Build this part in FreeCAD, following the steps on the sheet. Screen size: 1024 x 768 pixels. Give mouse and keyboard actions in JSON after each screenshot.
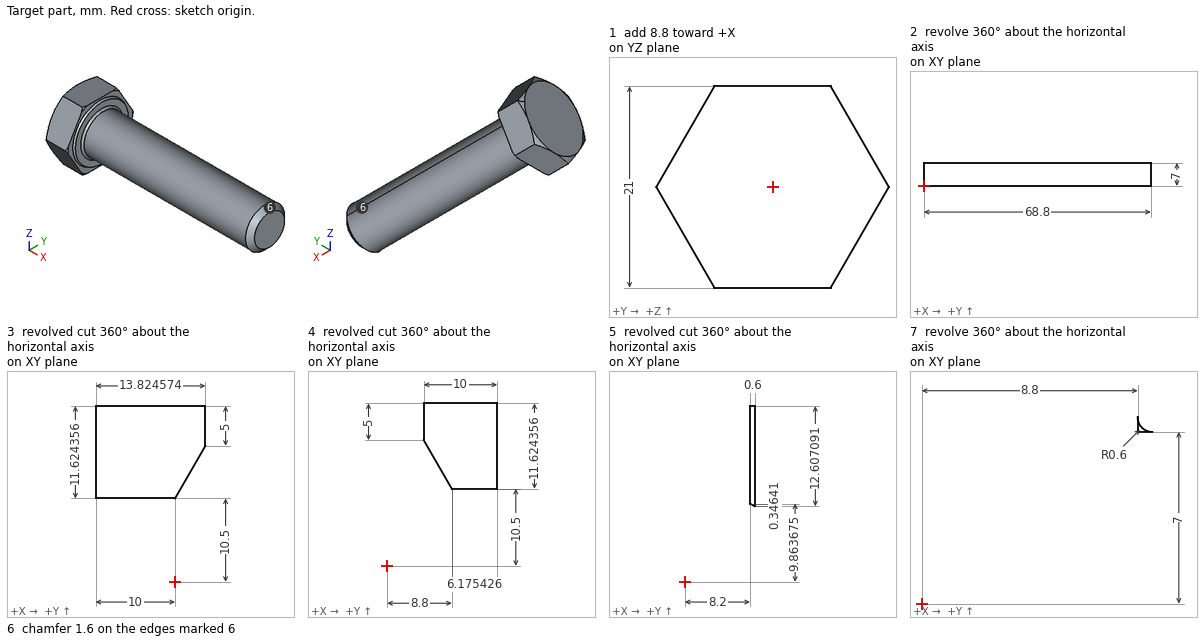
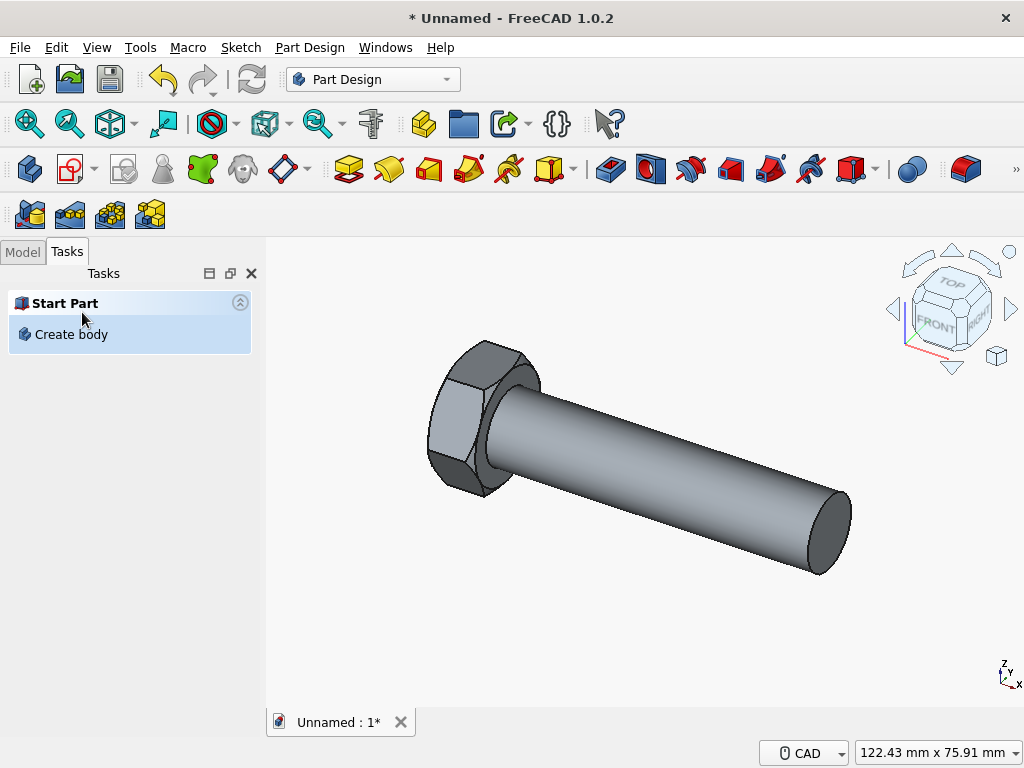
{"action": "left_click", "coordinate": [70, 170]}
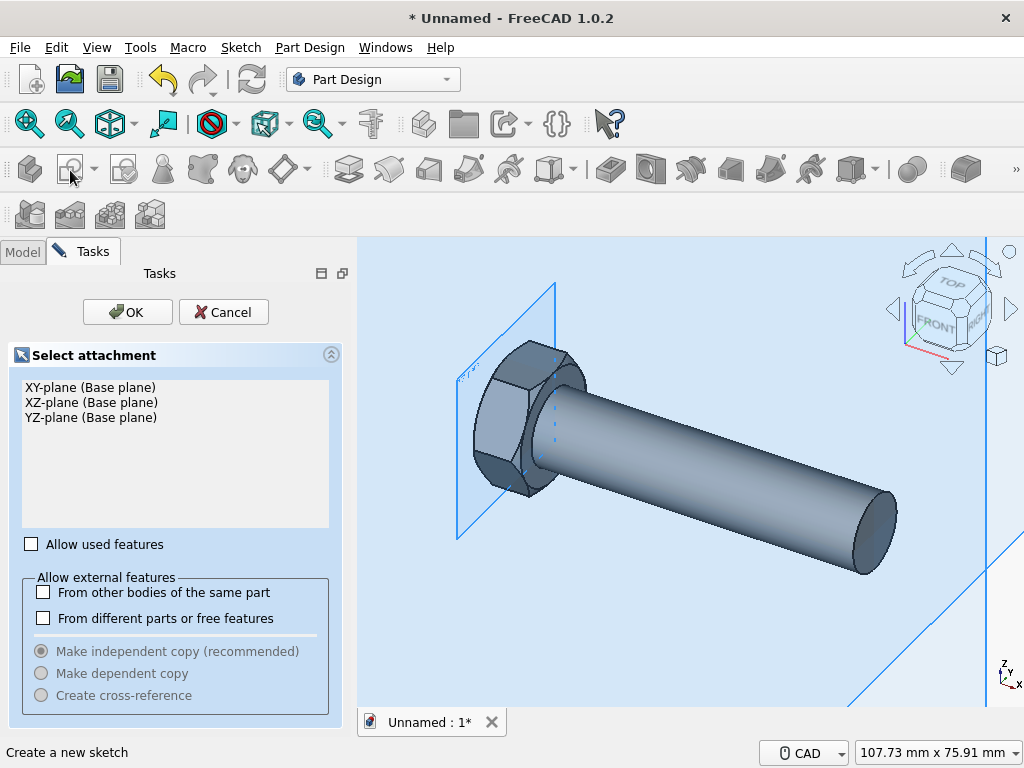
{"action": "left_click", "coordinate": [82, 388]}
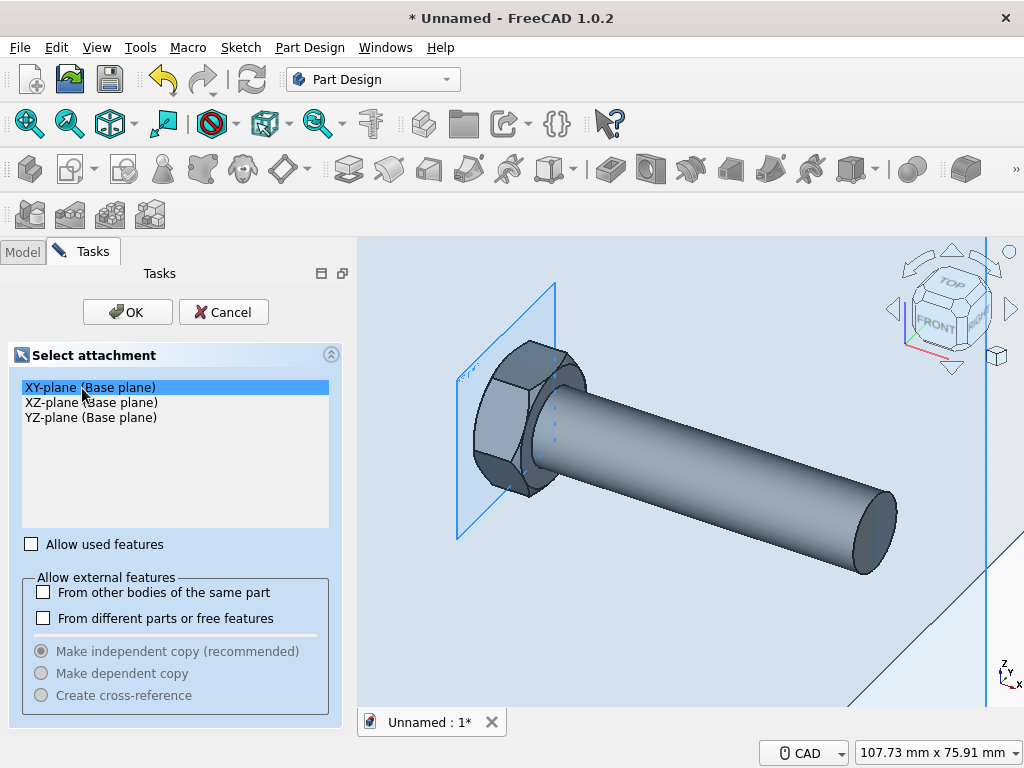
{"action": "left_click", "coordinate": [128, 312]}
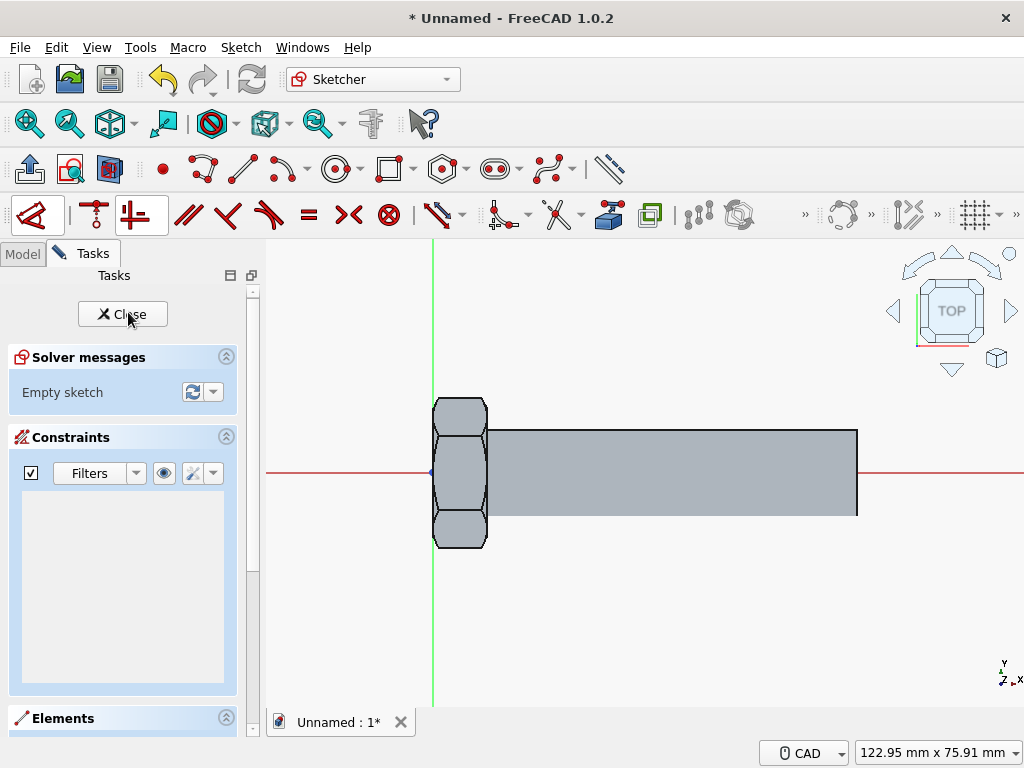
{"action": "left_click", "coordinate": [110, 170]}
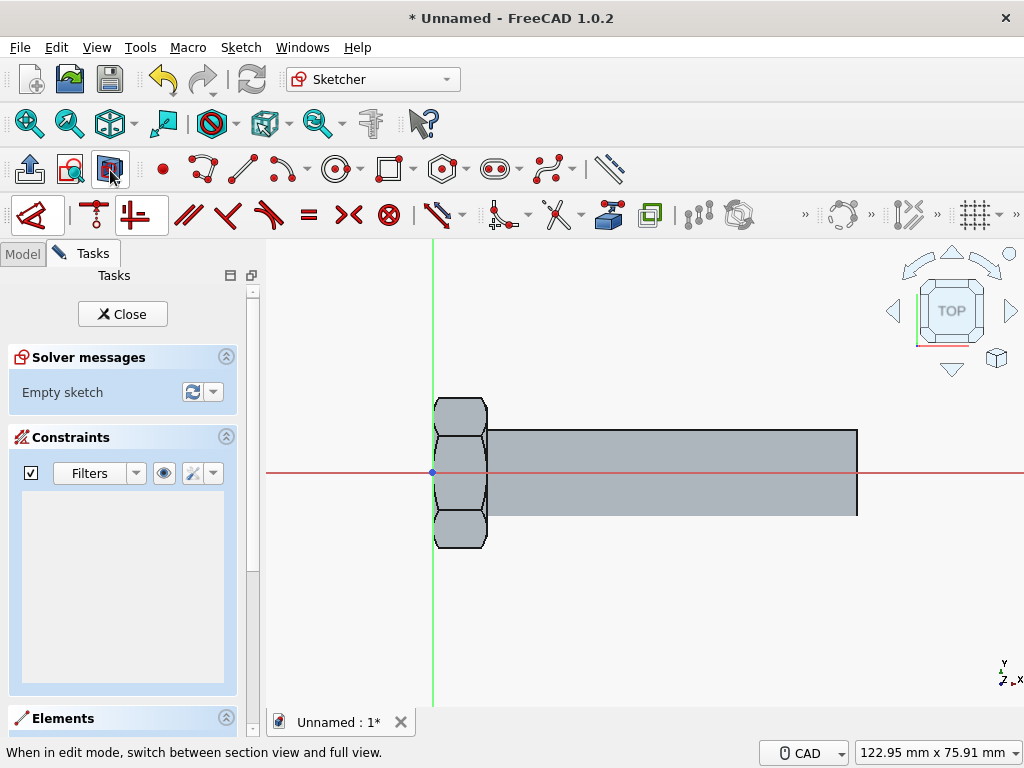
{"action": "scroll", "coordinate": [365, 349], "scroll_direction": "up", "scroll_amount": 4}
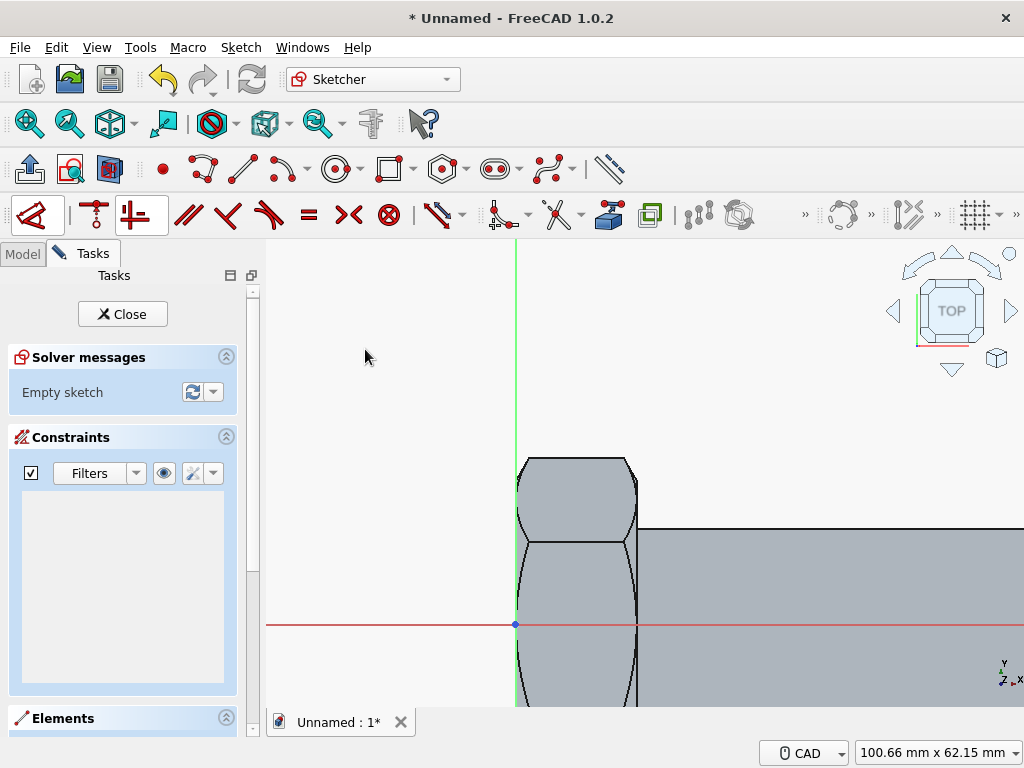
{"action": "left_click", "coordinate": [204, 170]}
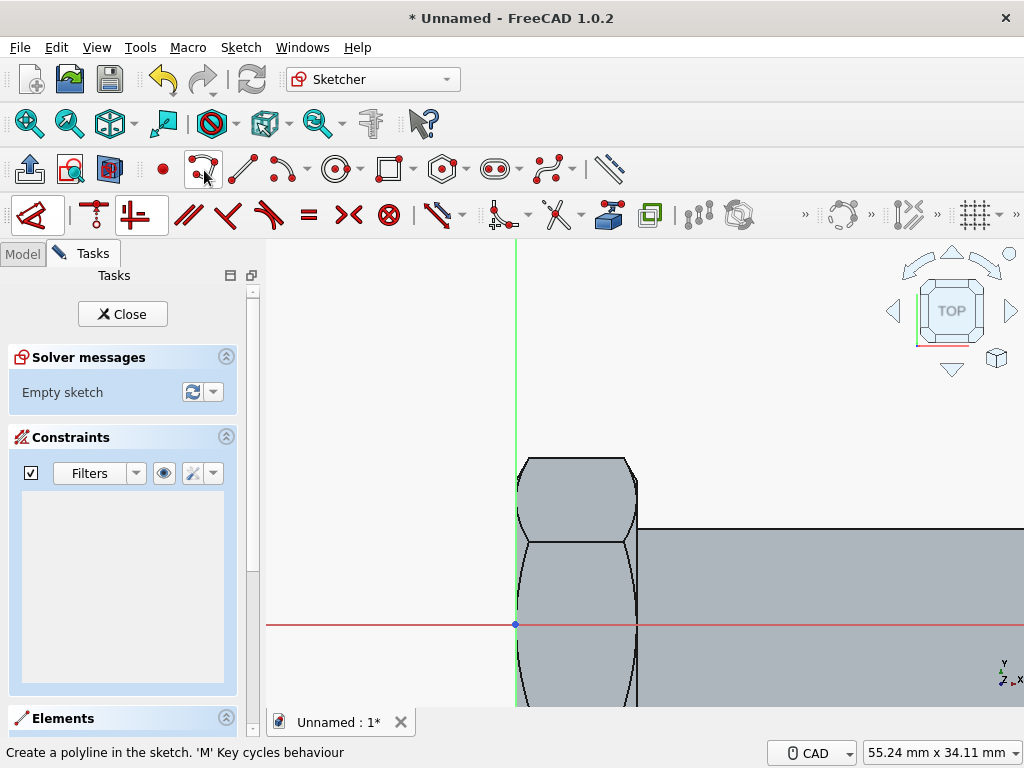
{"action": "left_click", "coordinate": [629, 489]}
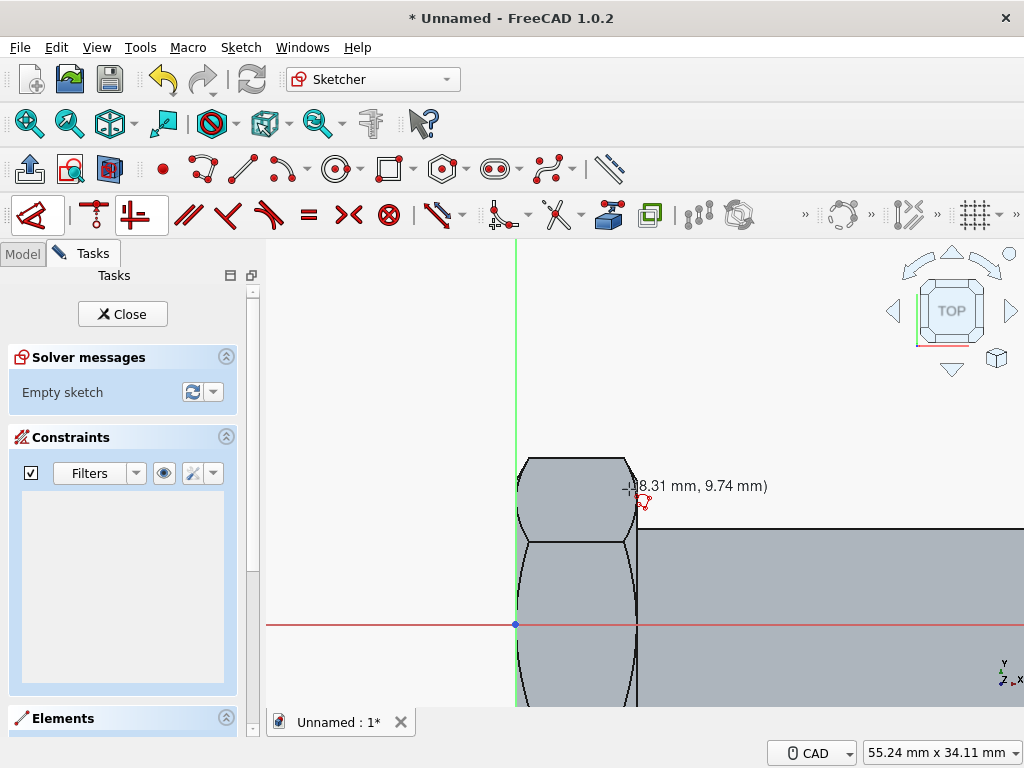
{"action": "scroll", "coordinate": [637, 494], "scroll_direction": "up", "scroll_amount": 3}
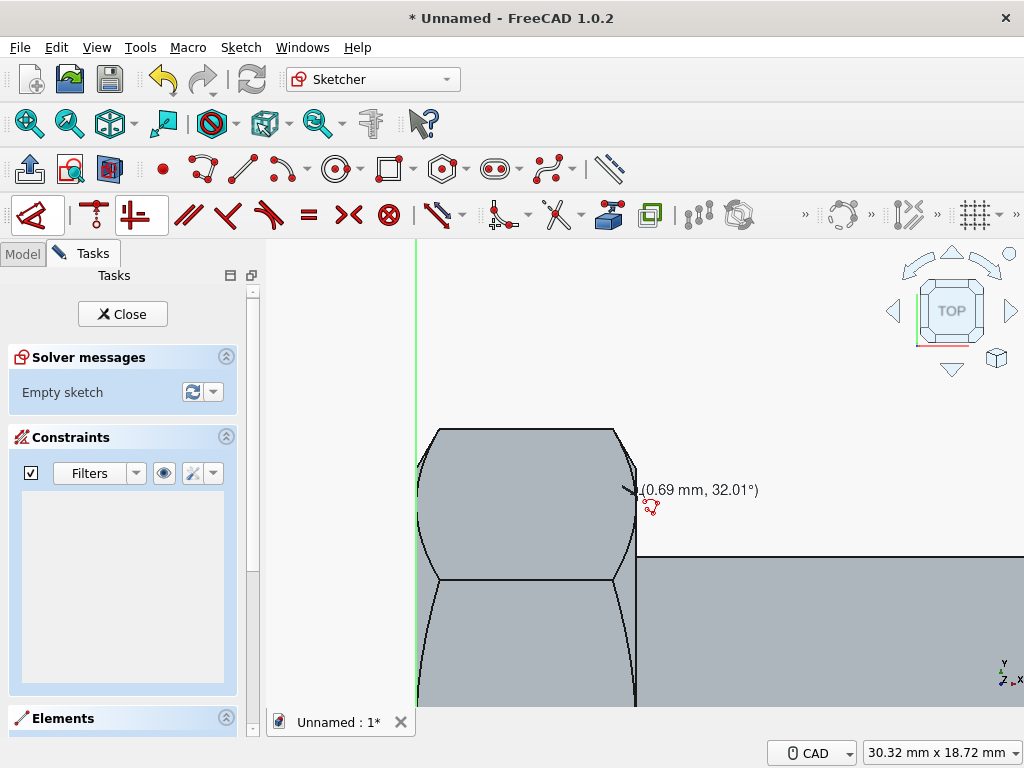
{"action": "left_click", "coordinate": [636, 494]}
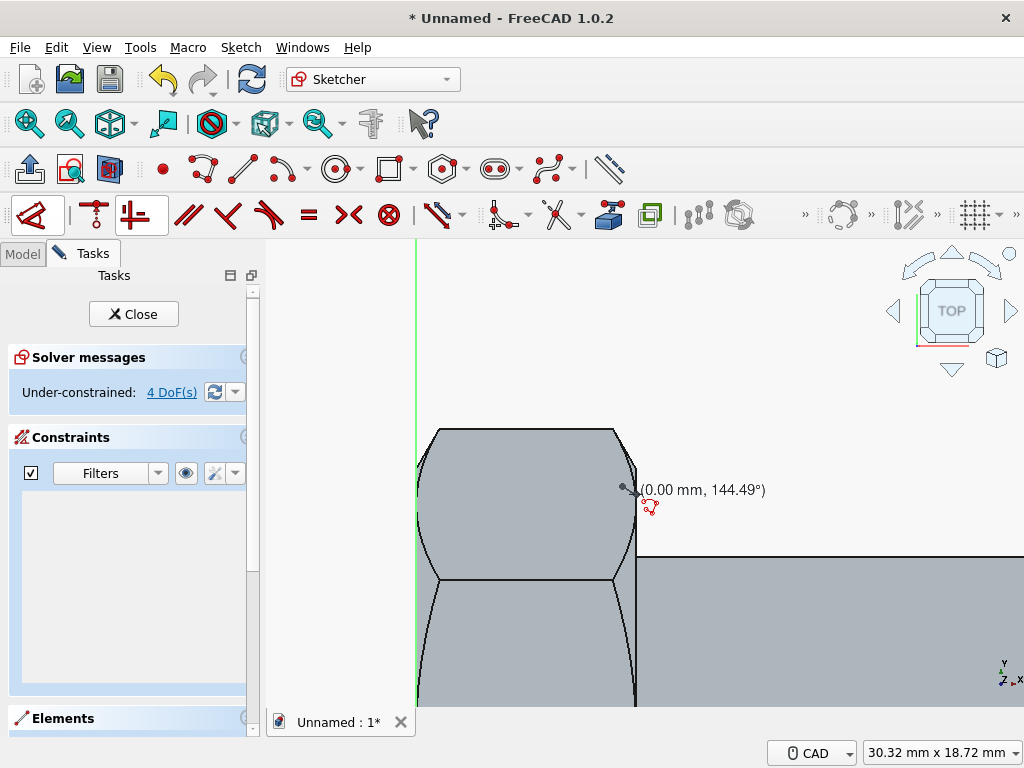
{"action": "scroll", "coordinate": [638, 495], "scroll_direction": "down", "scroll_amount": 3}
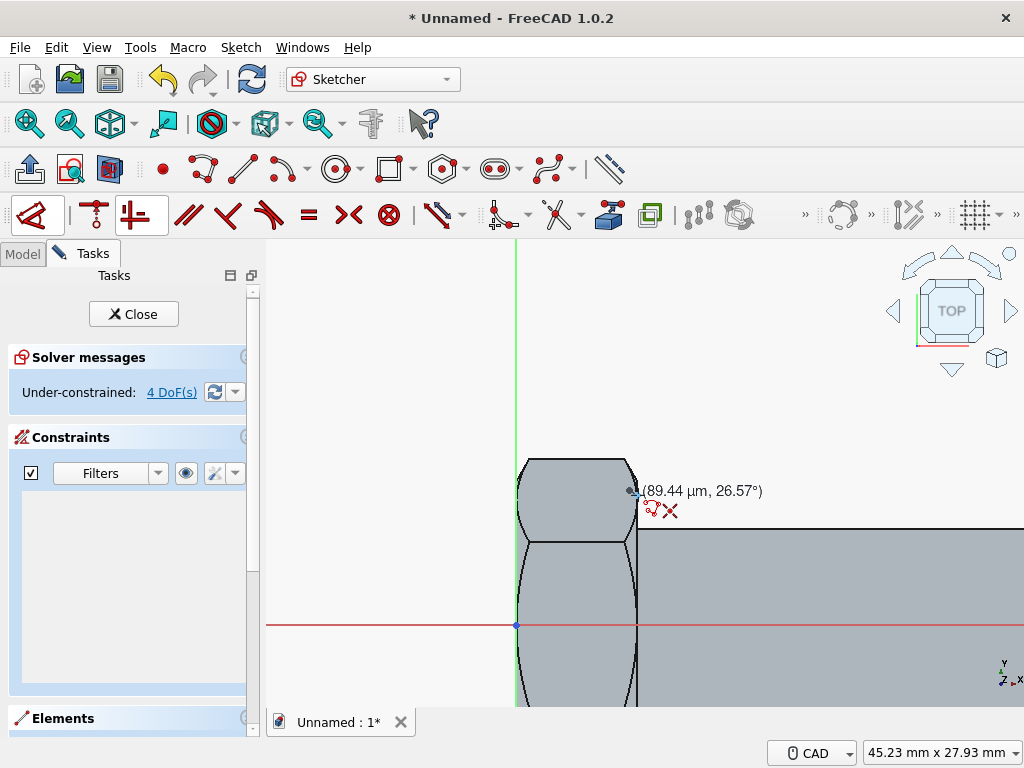
{"action": "left_click", "coordinate": [637, 322]}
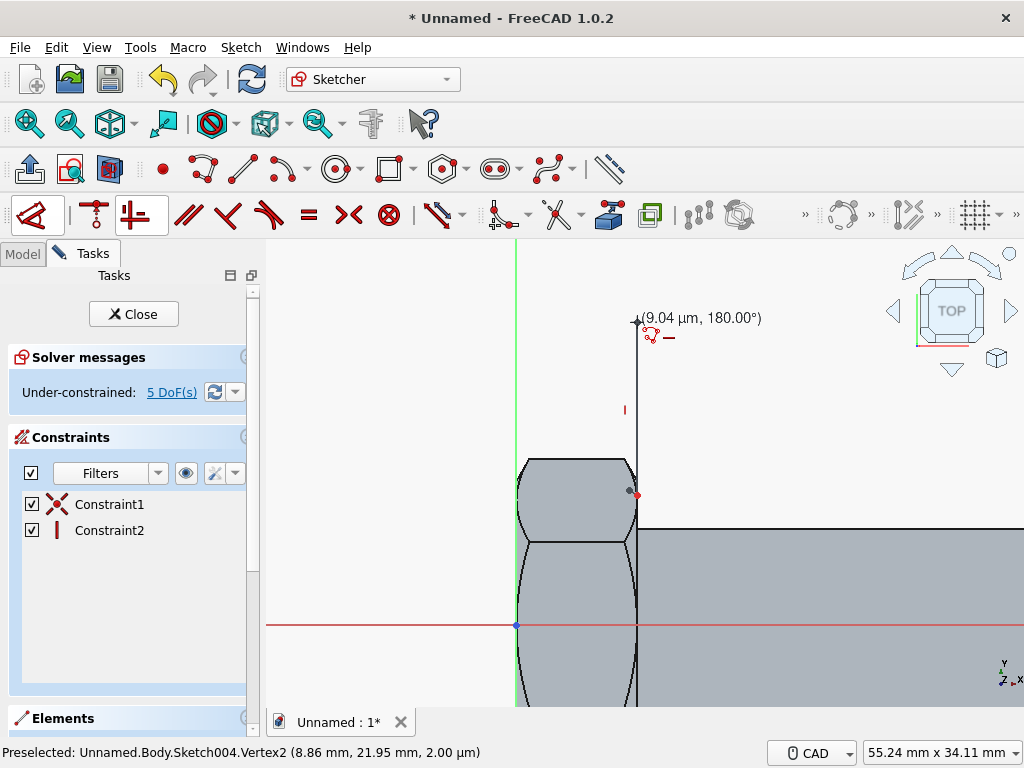
{"action": "scroll", "coordinate": [629, 322], "scroll_direction": "up", "scroll_amount": 4}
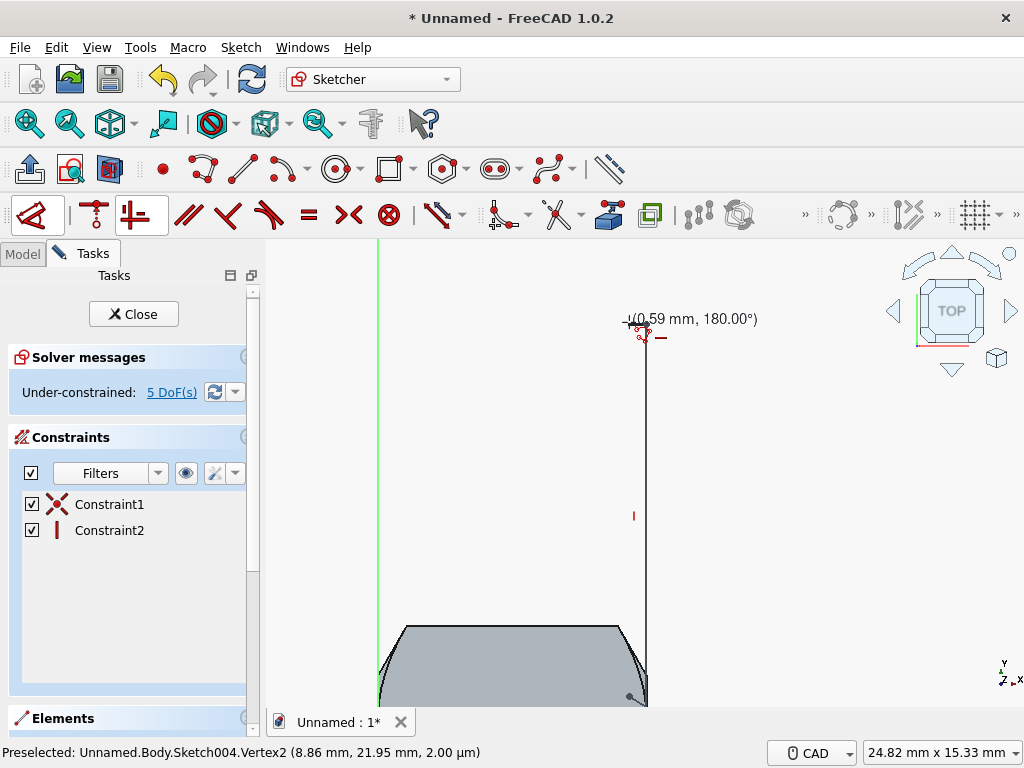
{"action": "left_click", "coordinate": [628, 322]}